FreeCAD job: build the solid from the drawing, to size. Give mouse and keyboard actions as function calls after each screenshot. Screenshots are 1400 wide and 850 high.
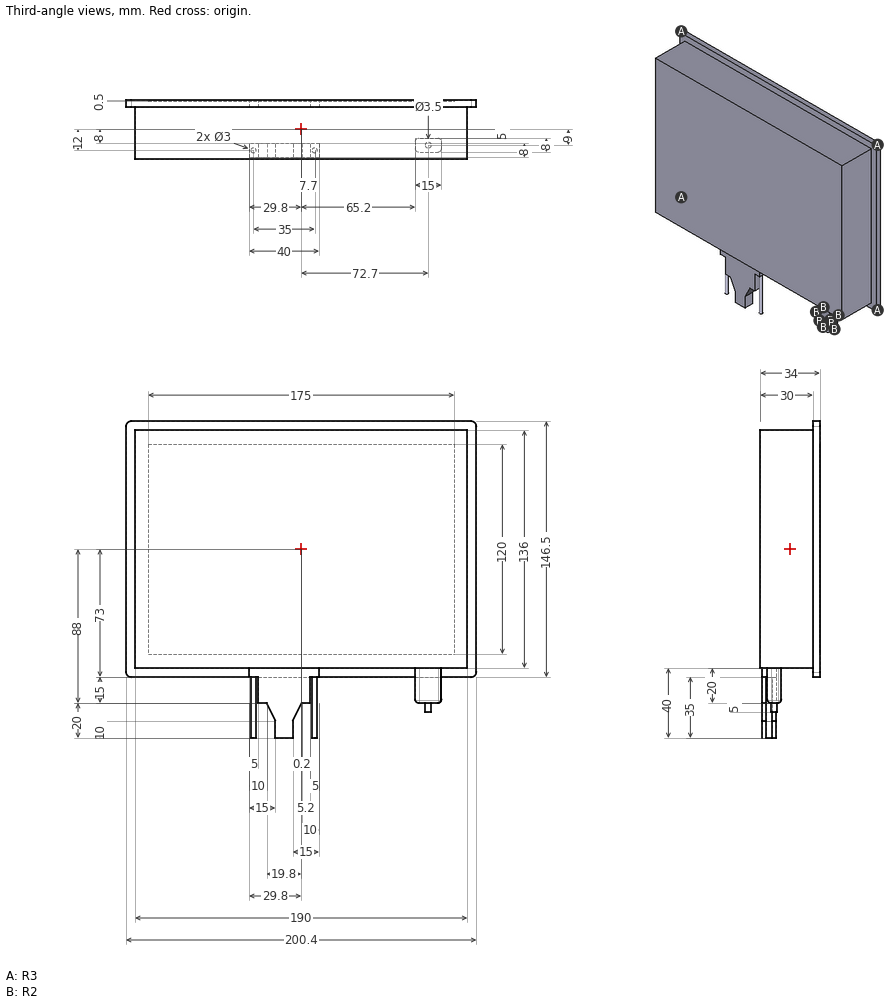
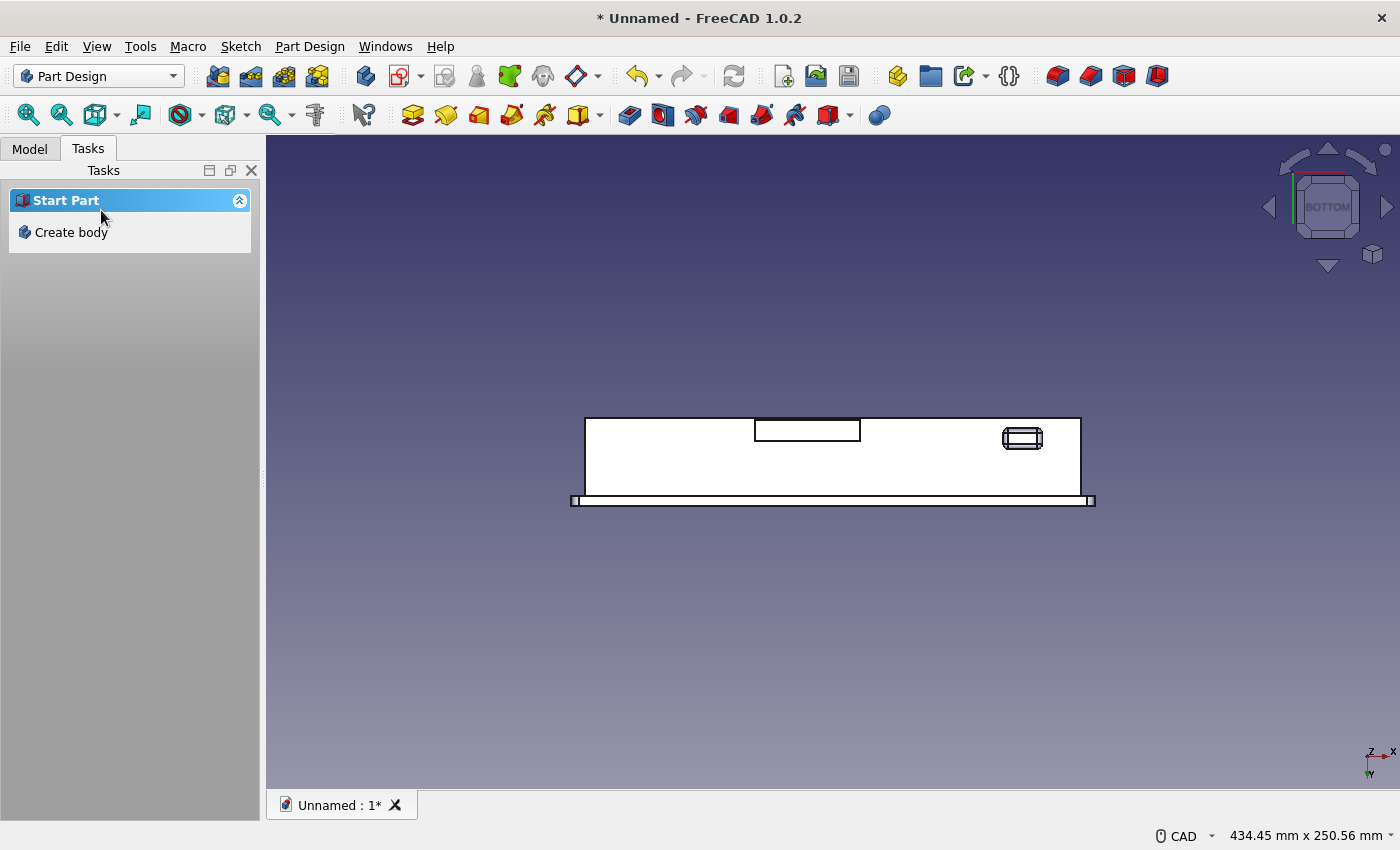
scroll(1031, 438, up, 5)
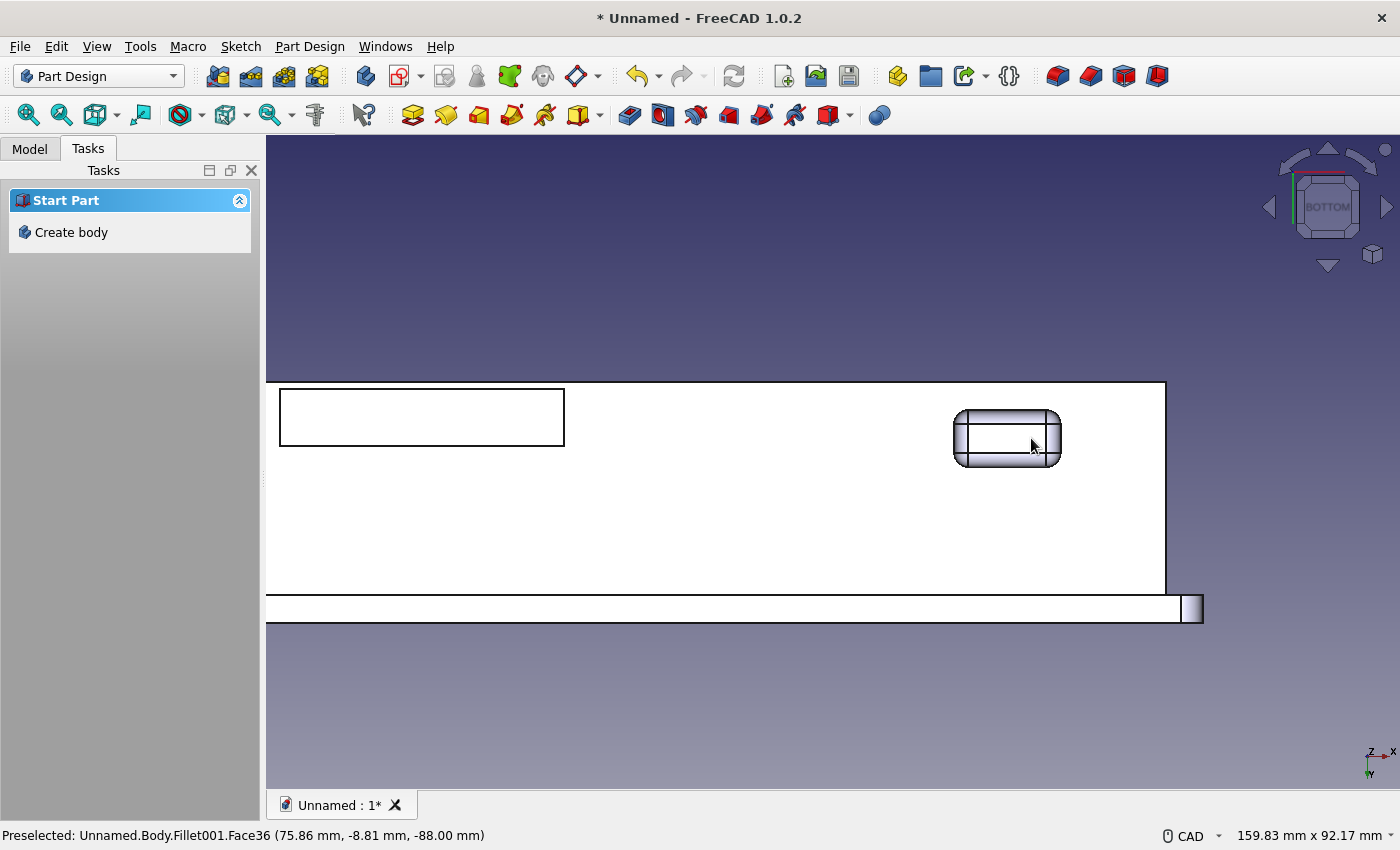
click(1030, 438)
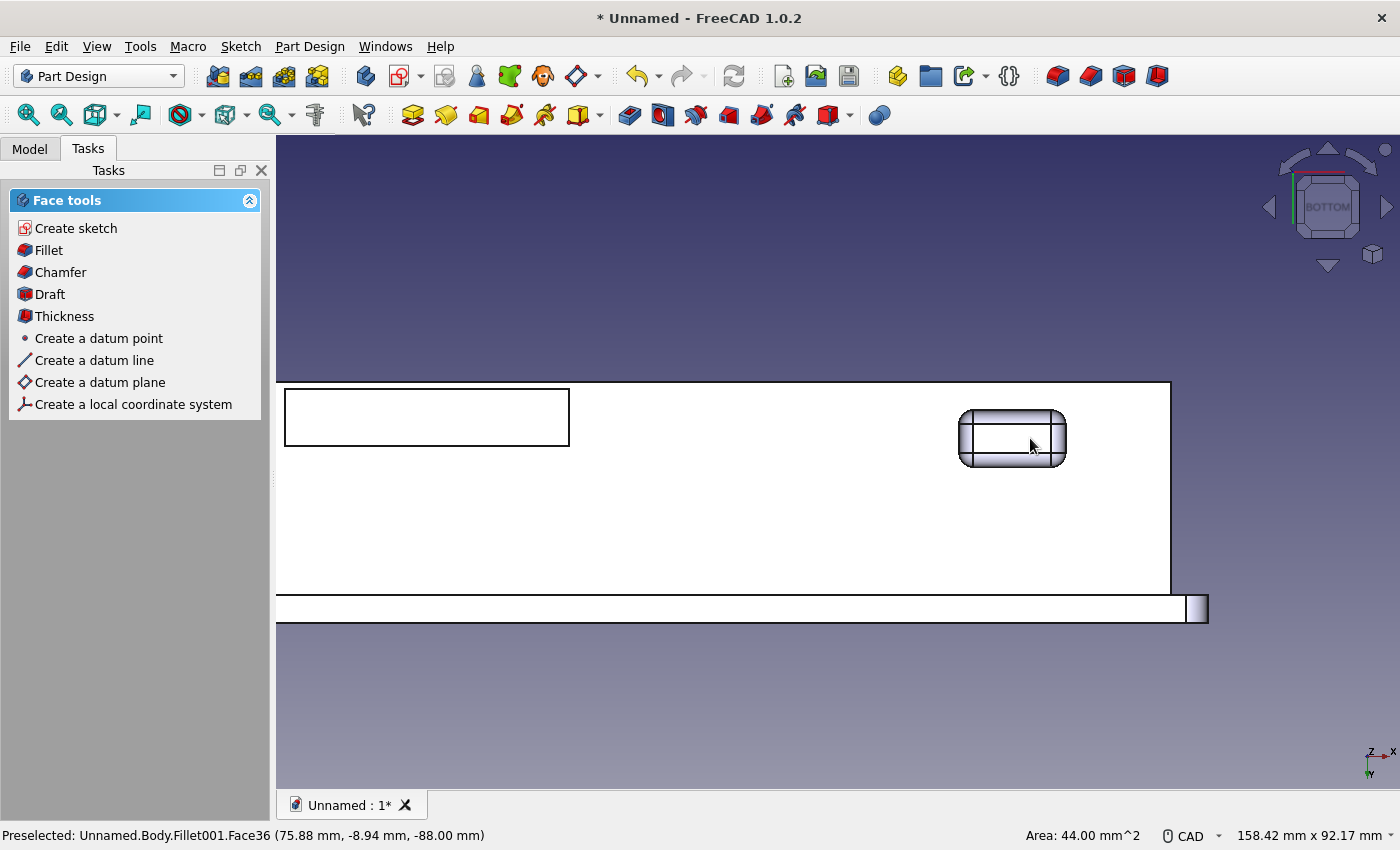
click(398, 76)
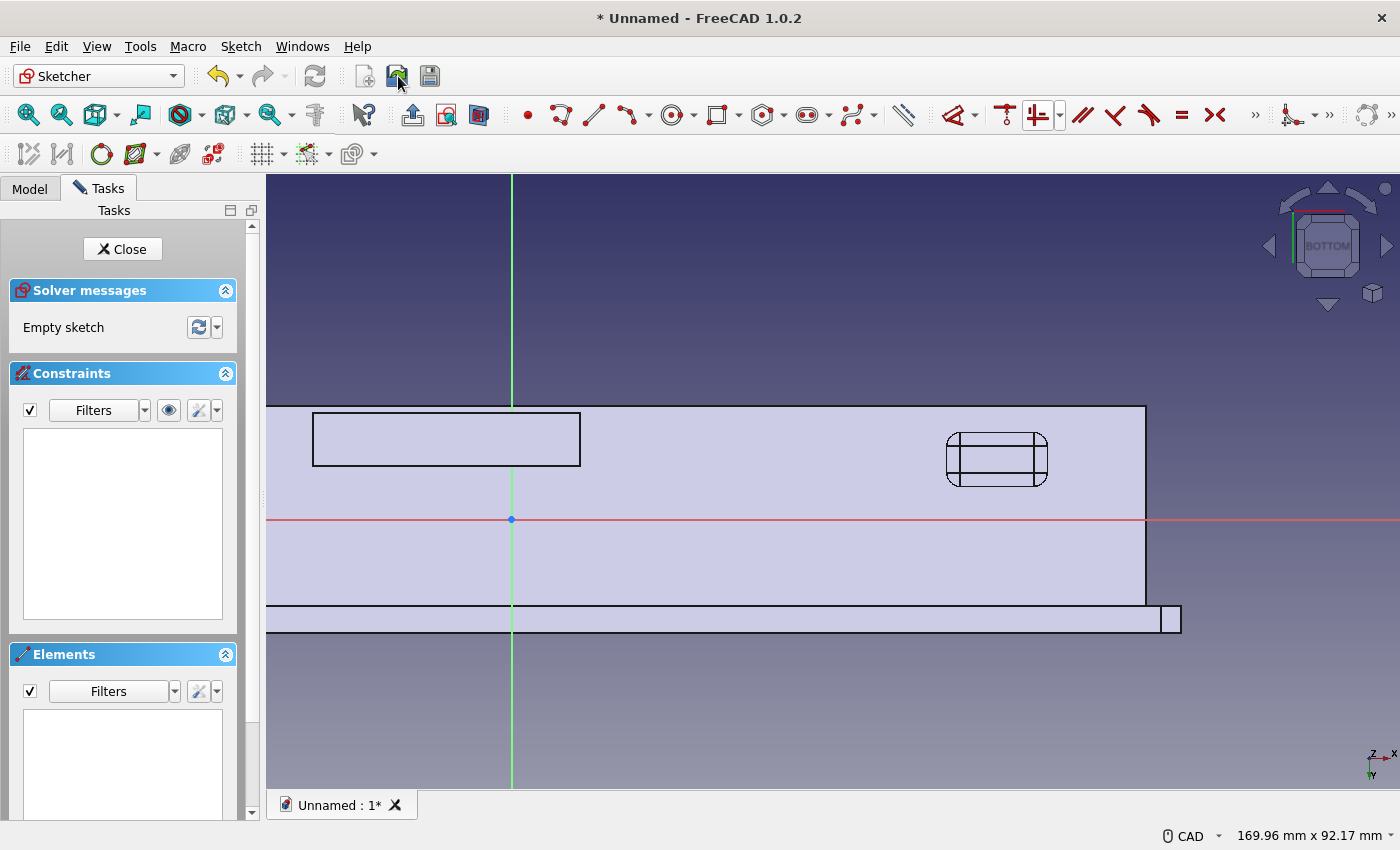
scroll(1012, 458, up, 14)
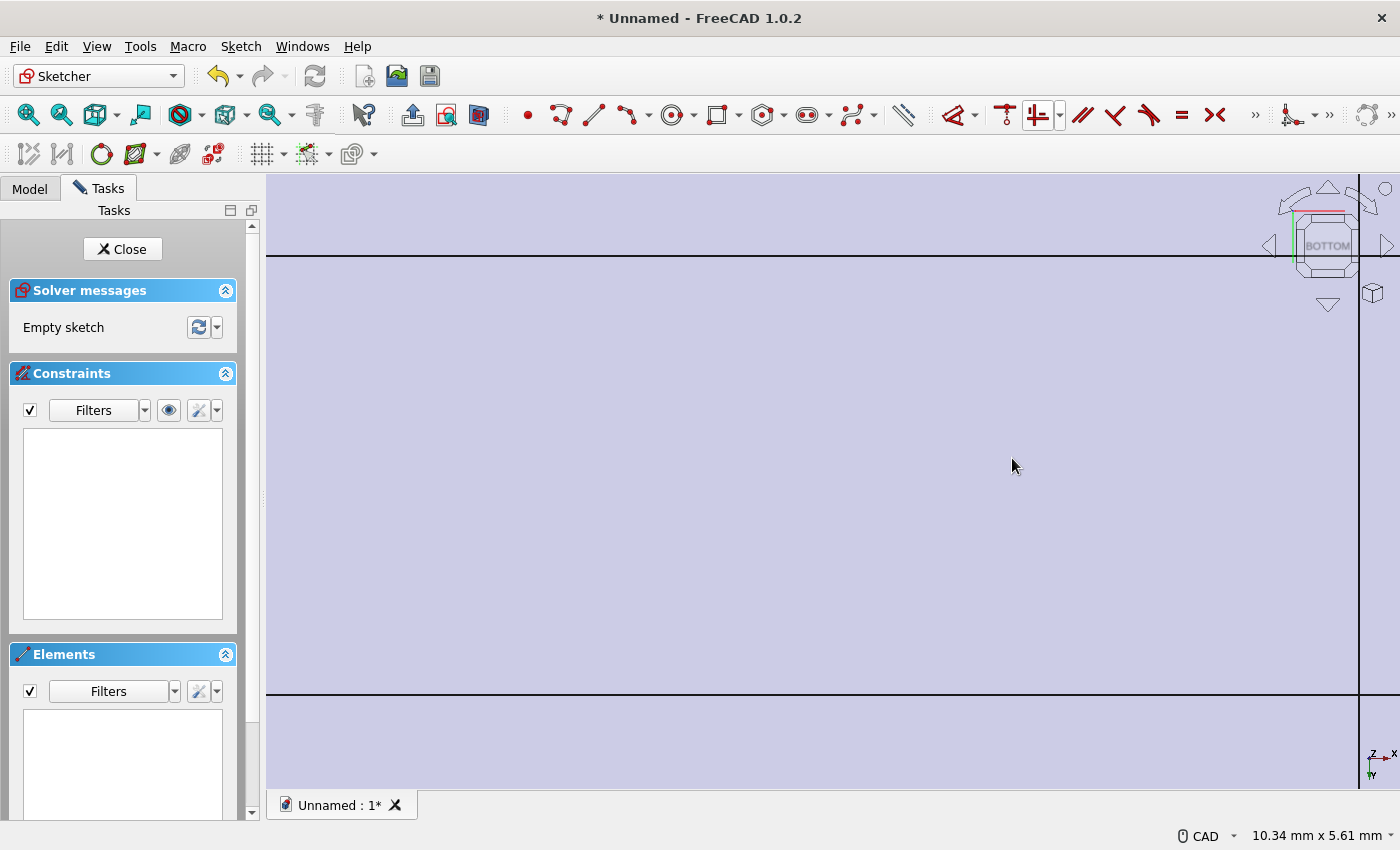
click(672, 116)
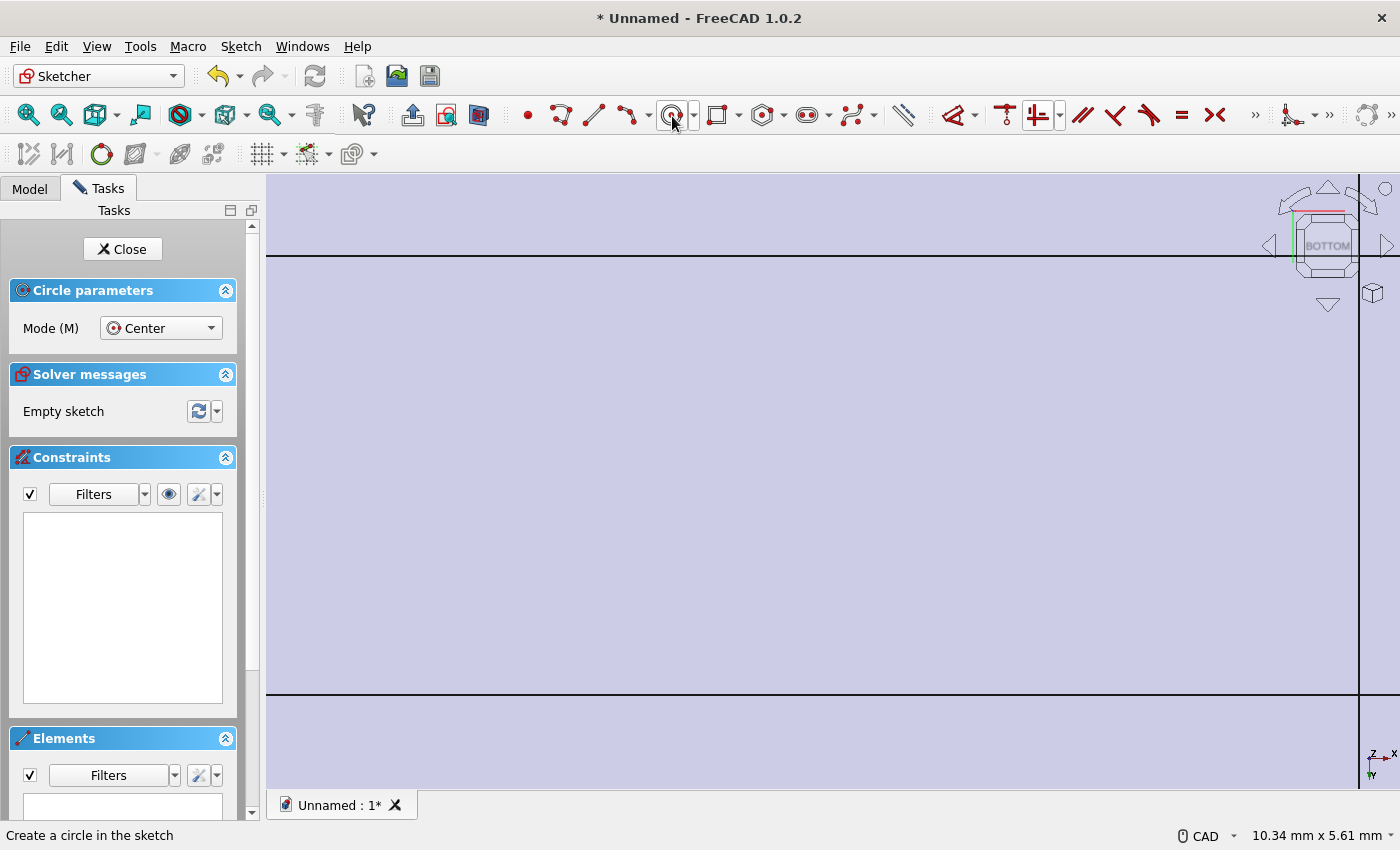
click(756, 475)
move(892, 339)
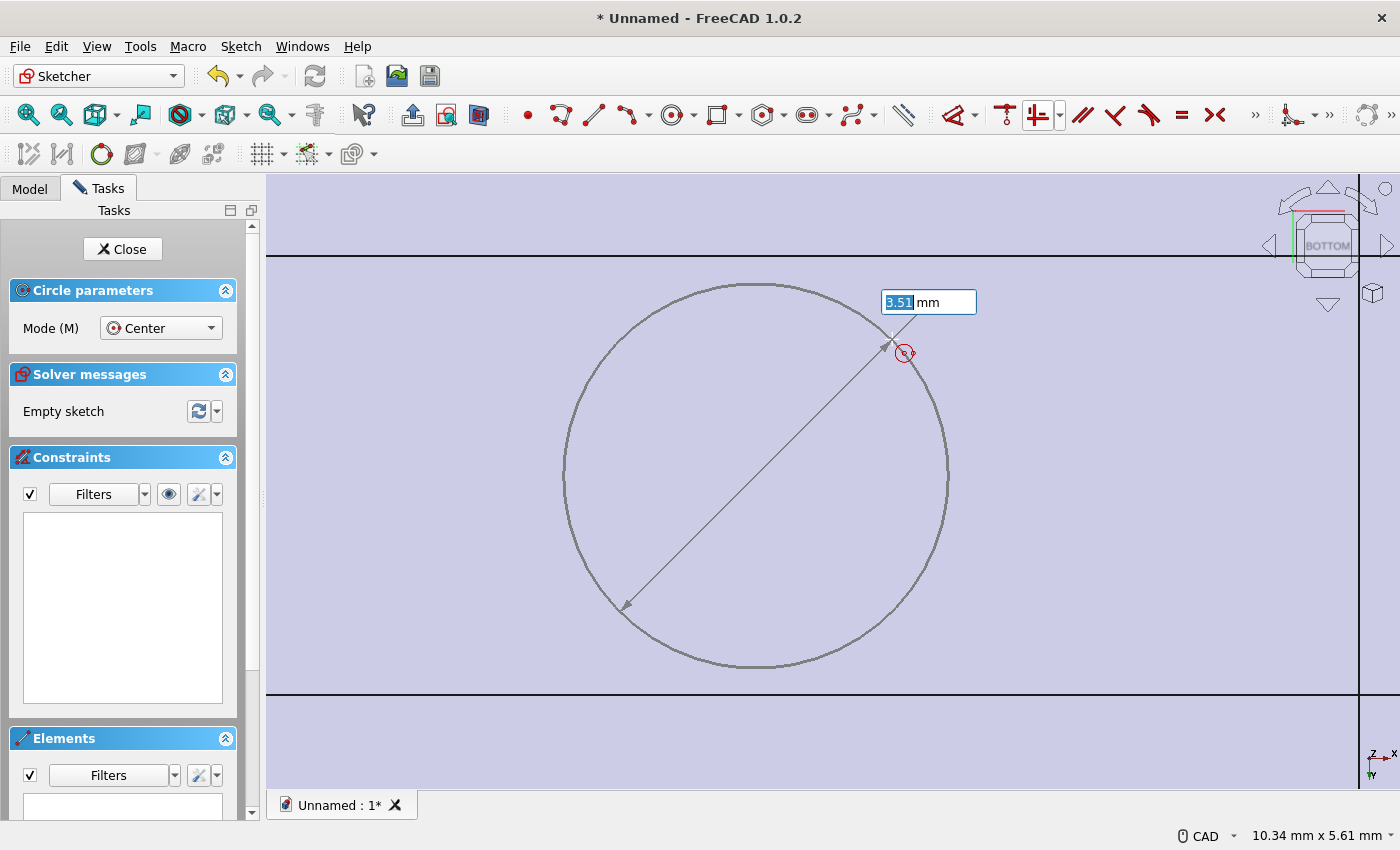
text(3.5)
key(Return)
key(Escape)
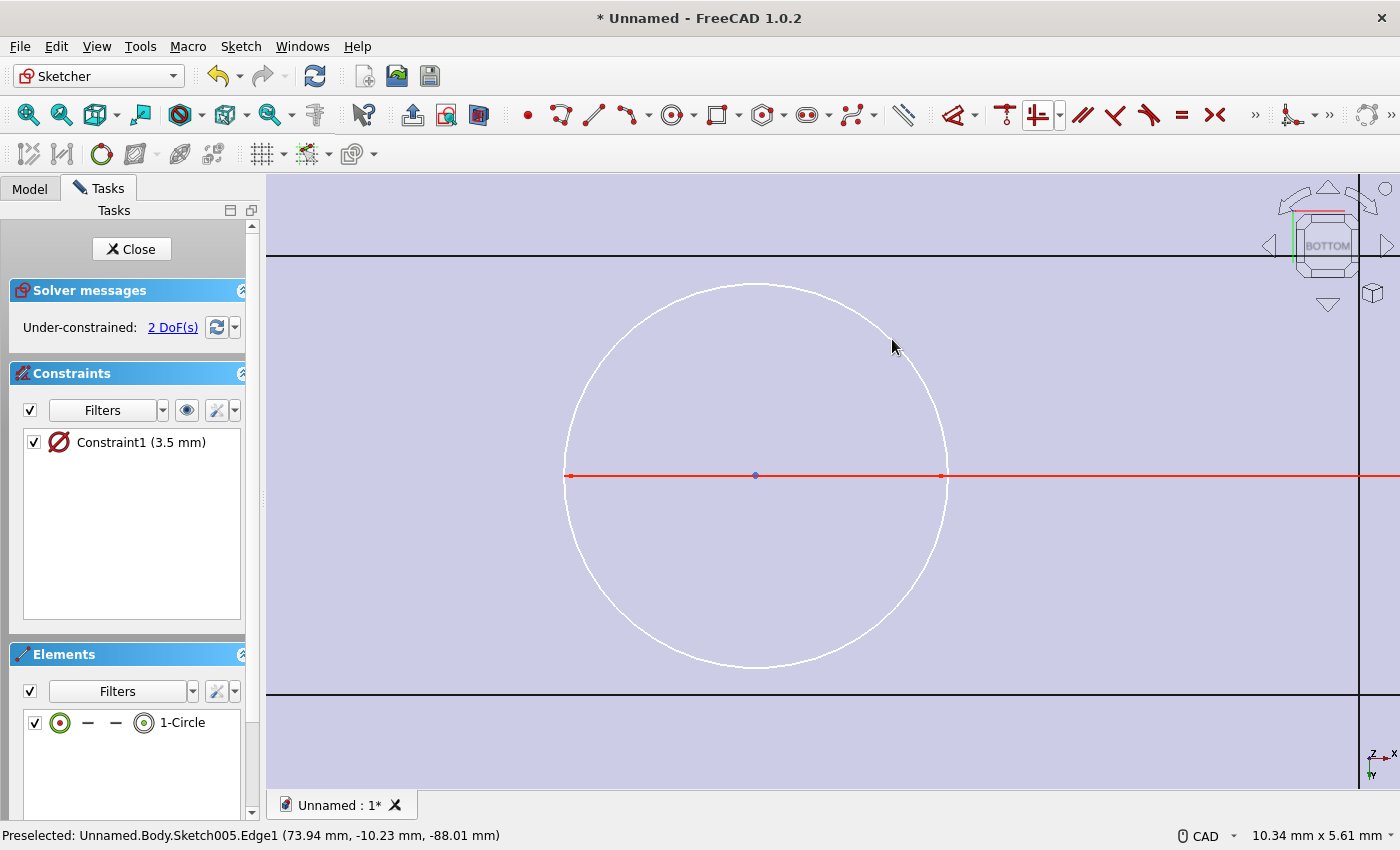
click(952, 116)